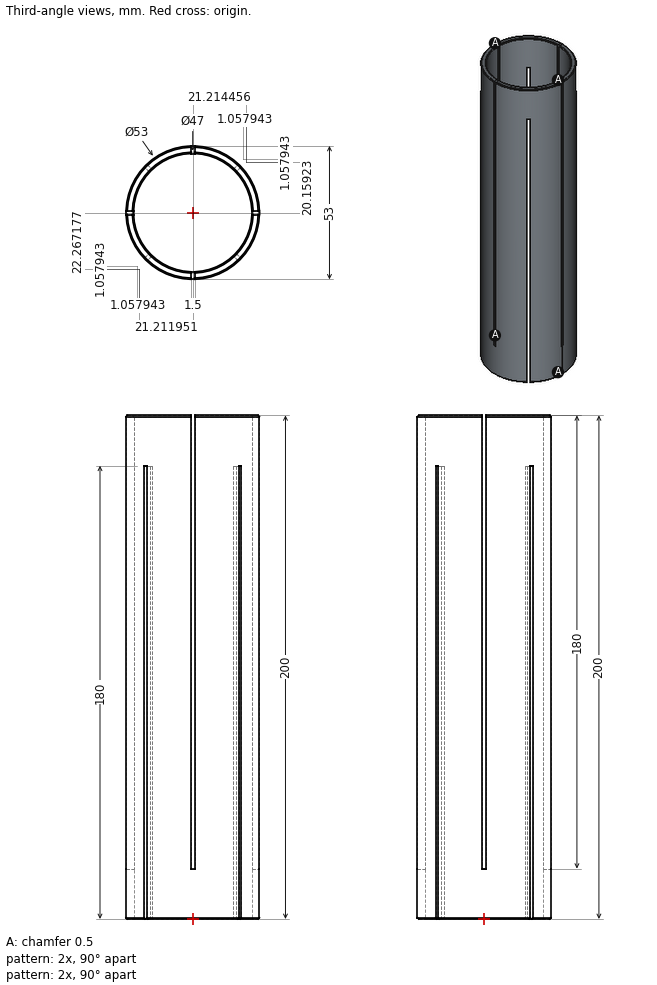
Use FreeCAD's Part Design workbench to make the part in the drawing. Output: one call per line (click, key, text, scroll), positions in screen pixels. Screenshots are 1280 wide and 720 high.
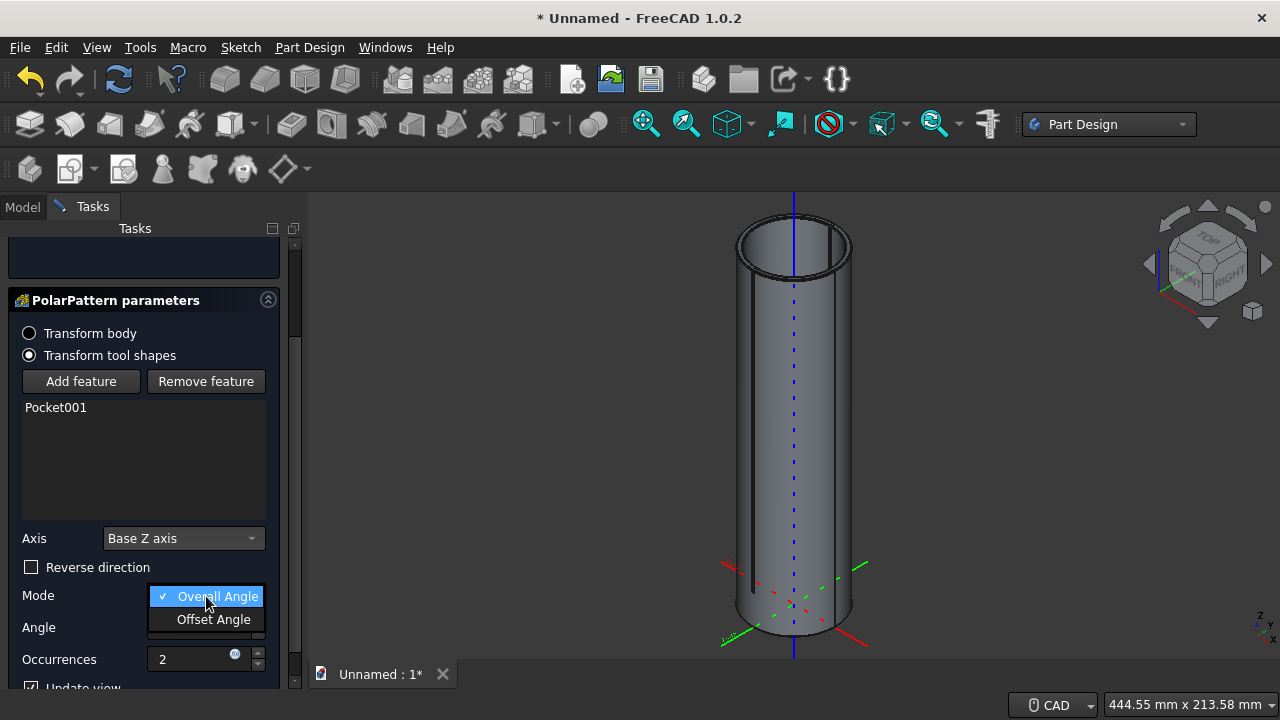
click(206, 620)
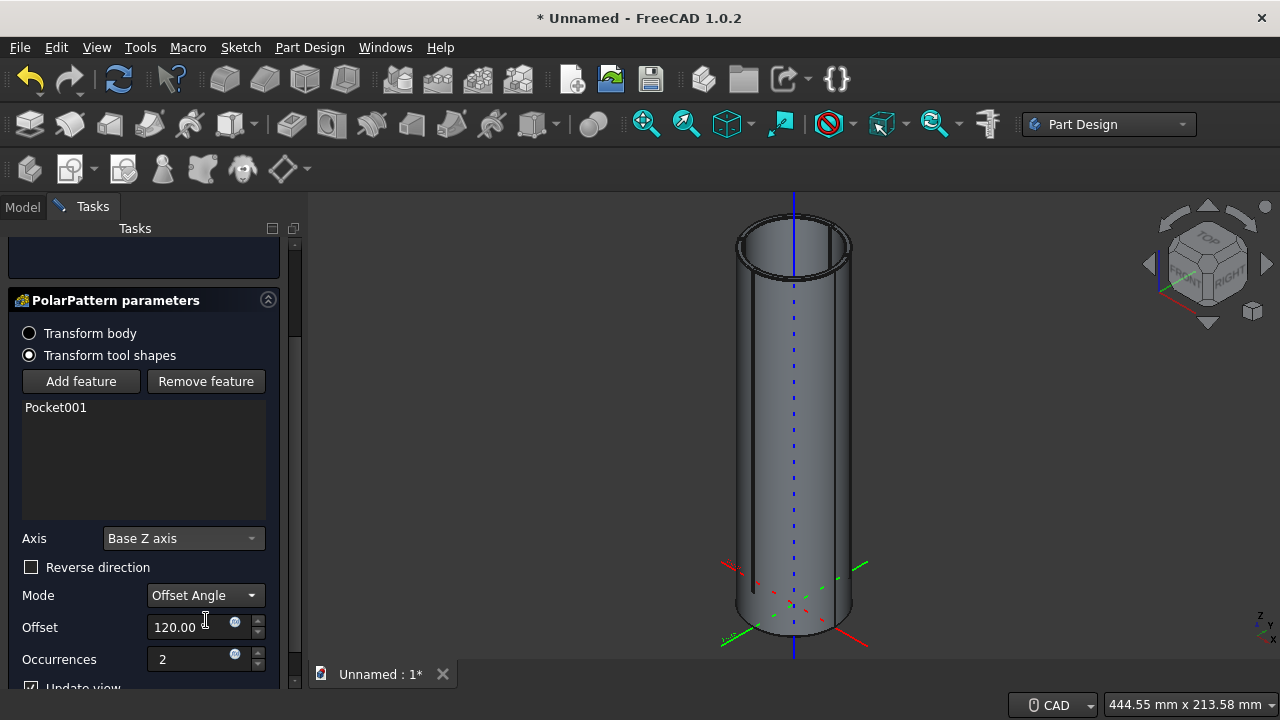
triple_click(198, 627)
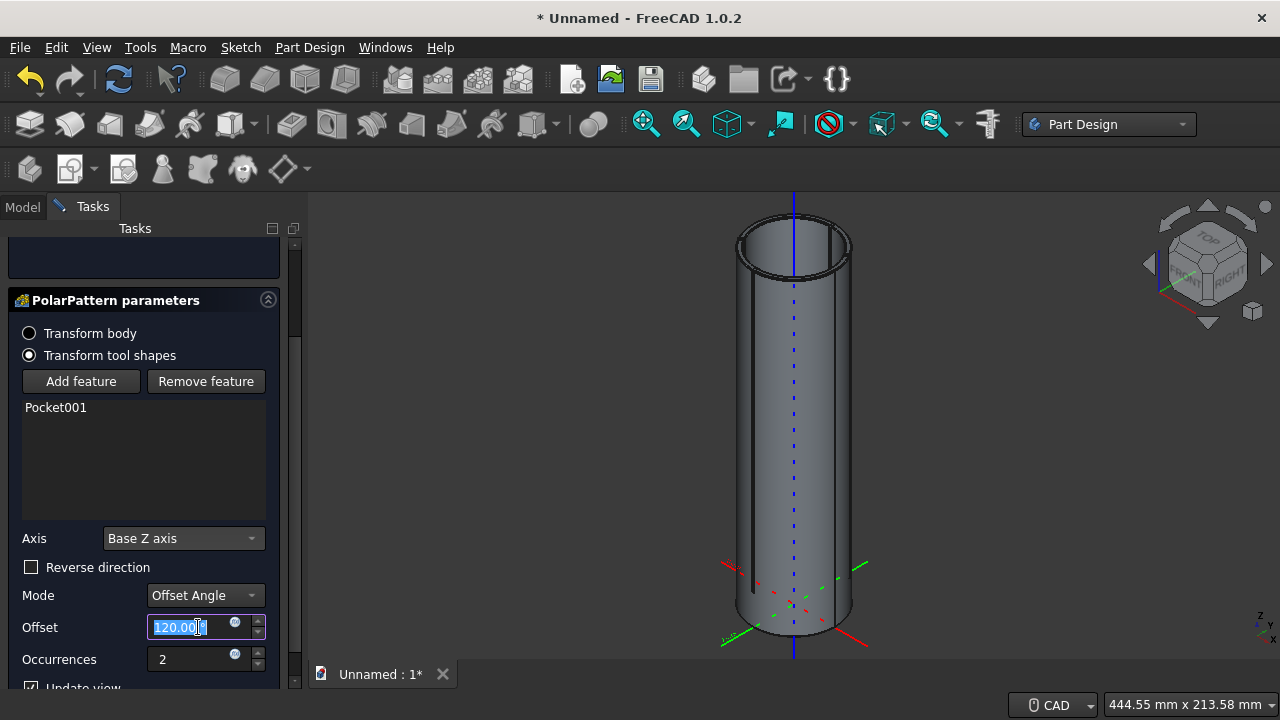
text(90)
key(Tab)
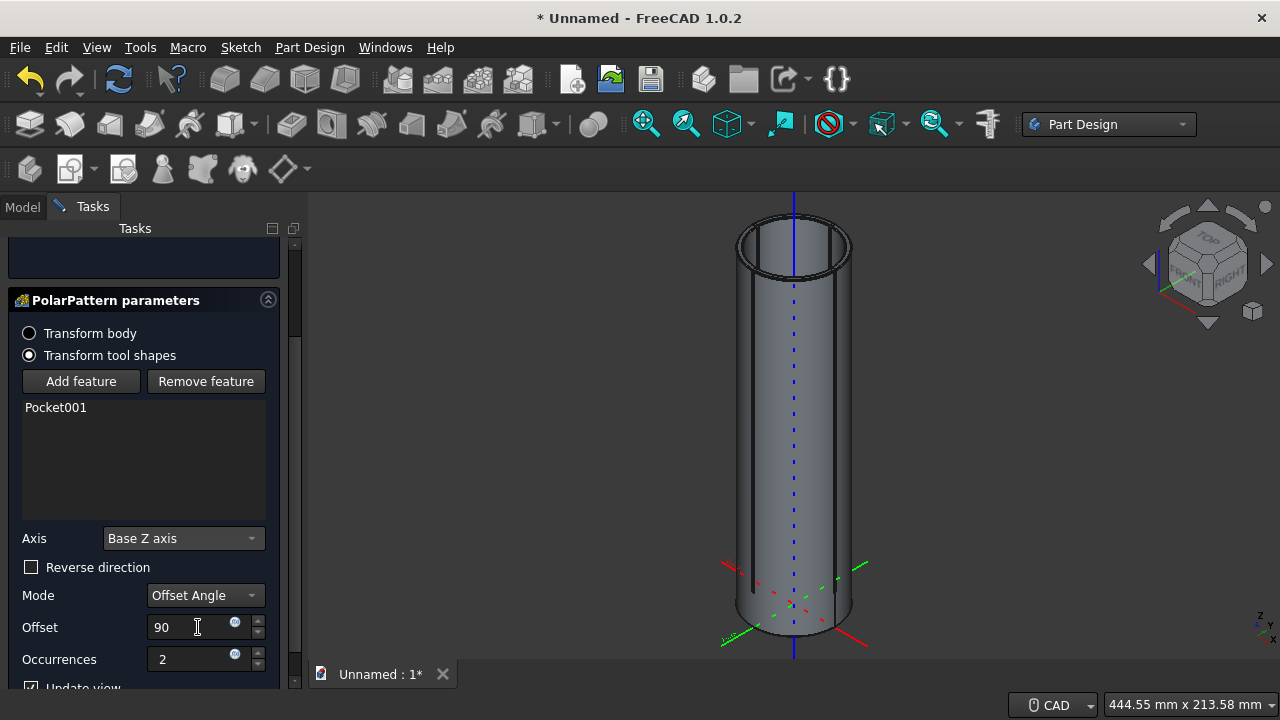
triple_click(198, 659)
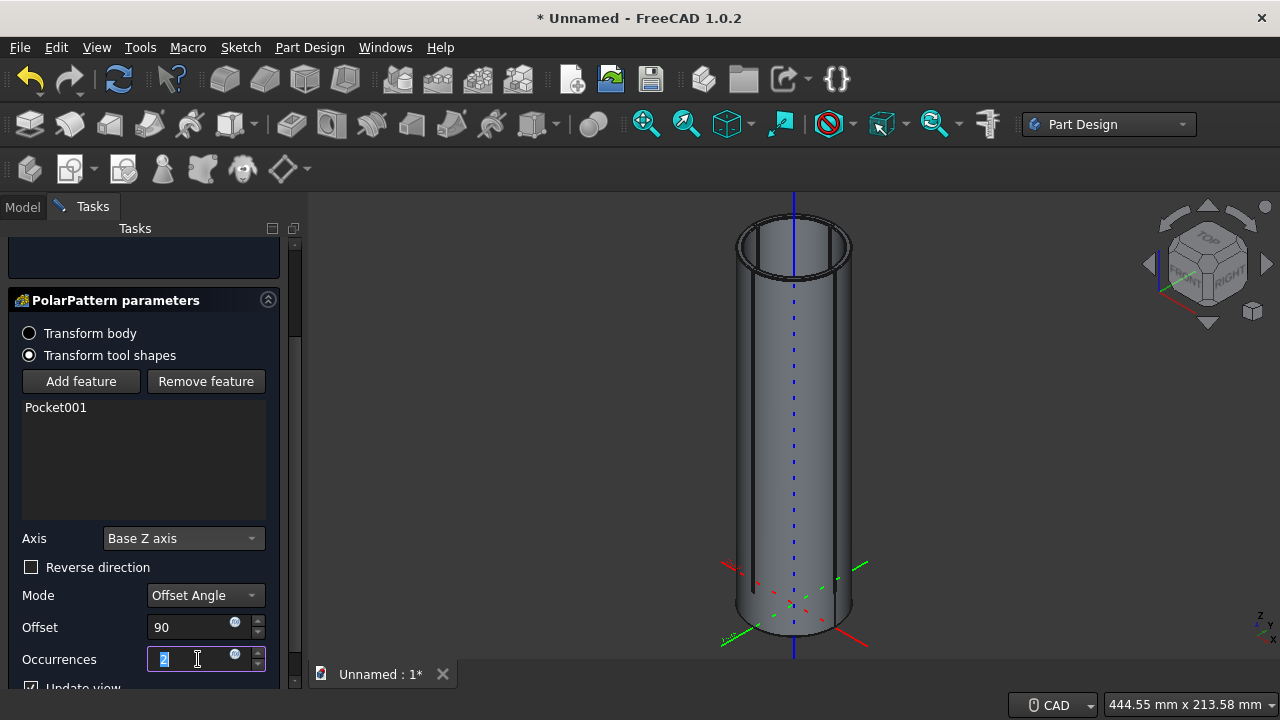
text(2)
key(Tab)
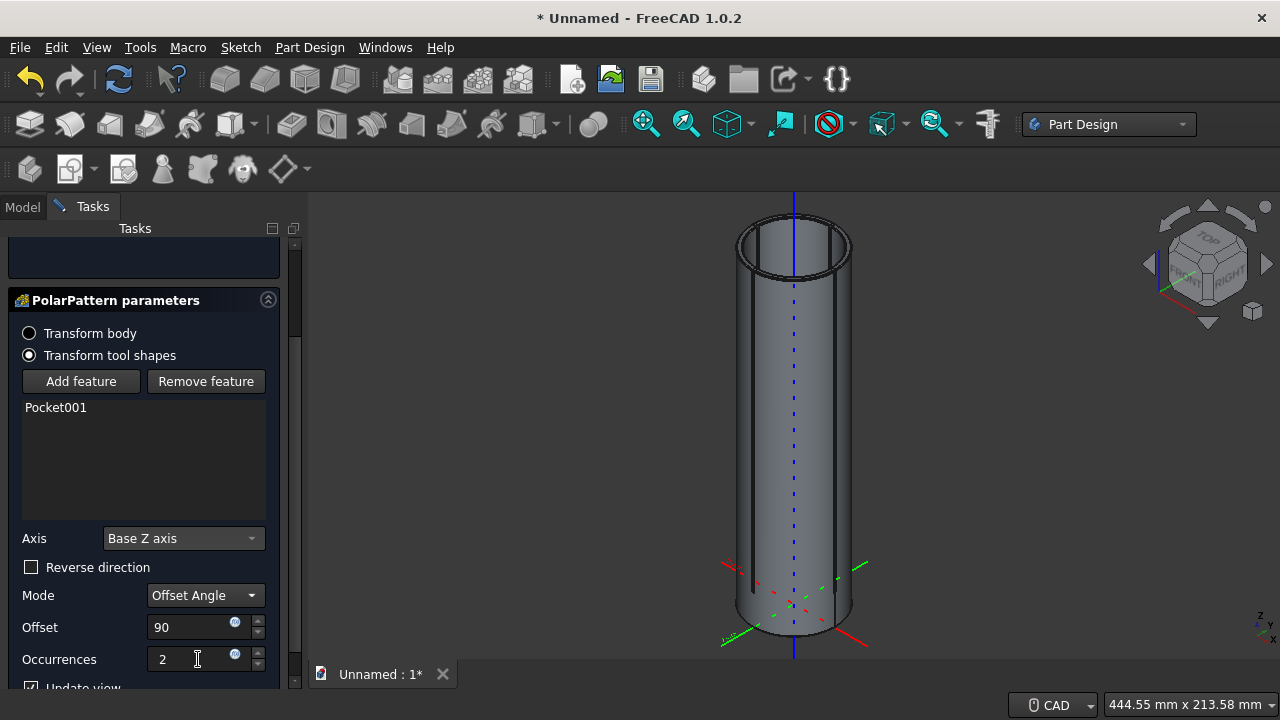
scroll(295, 463, up, 3)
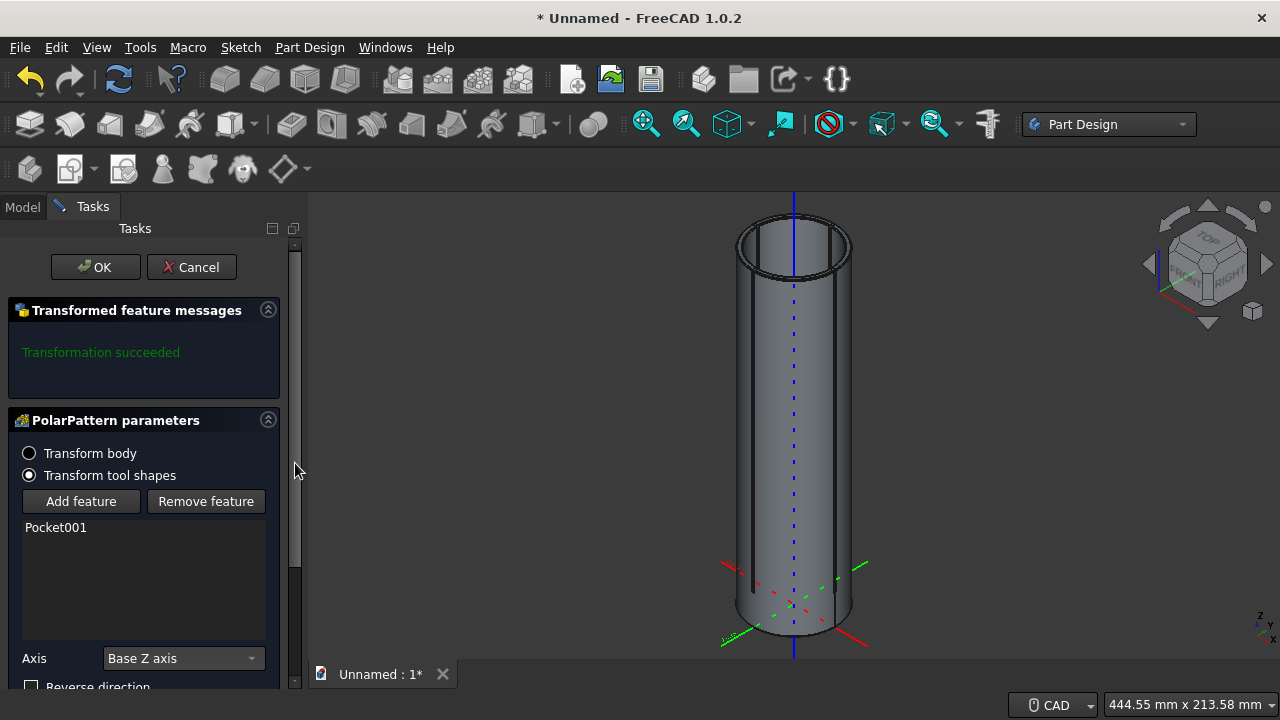
click(96, 267)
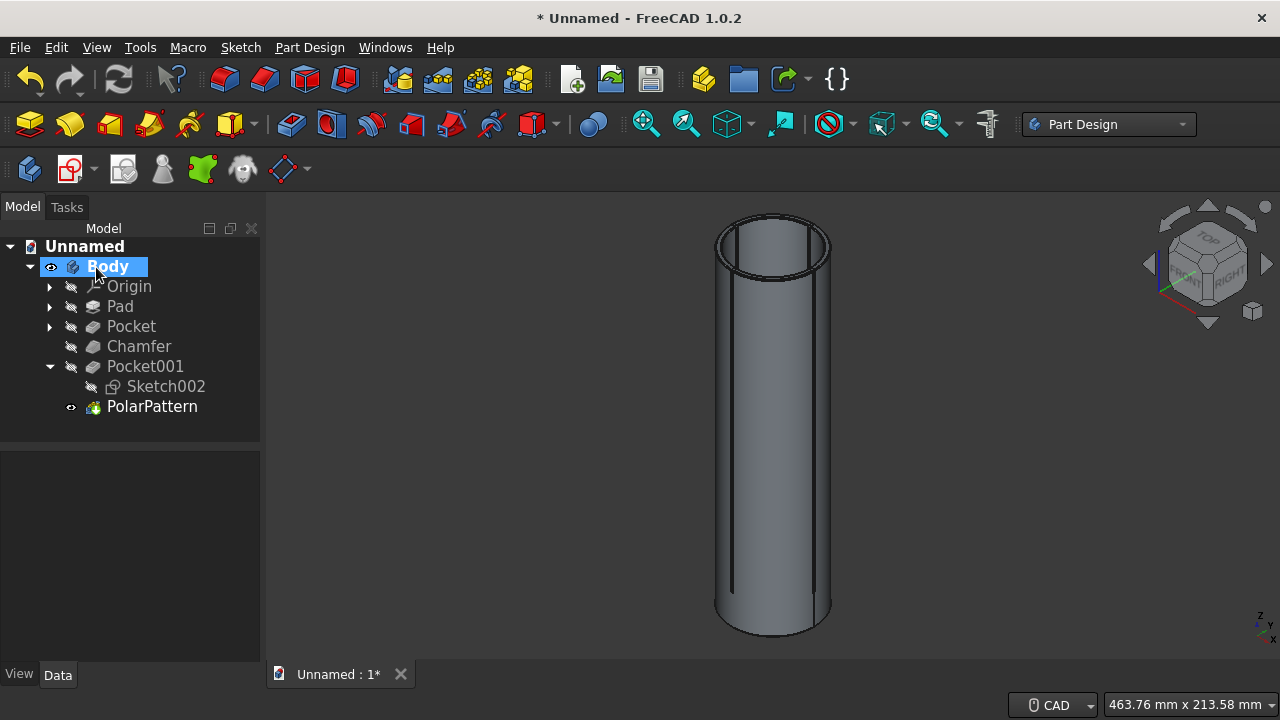
key(5)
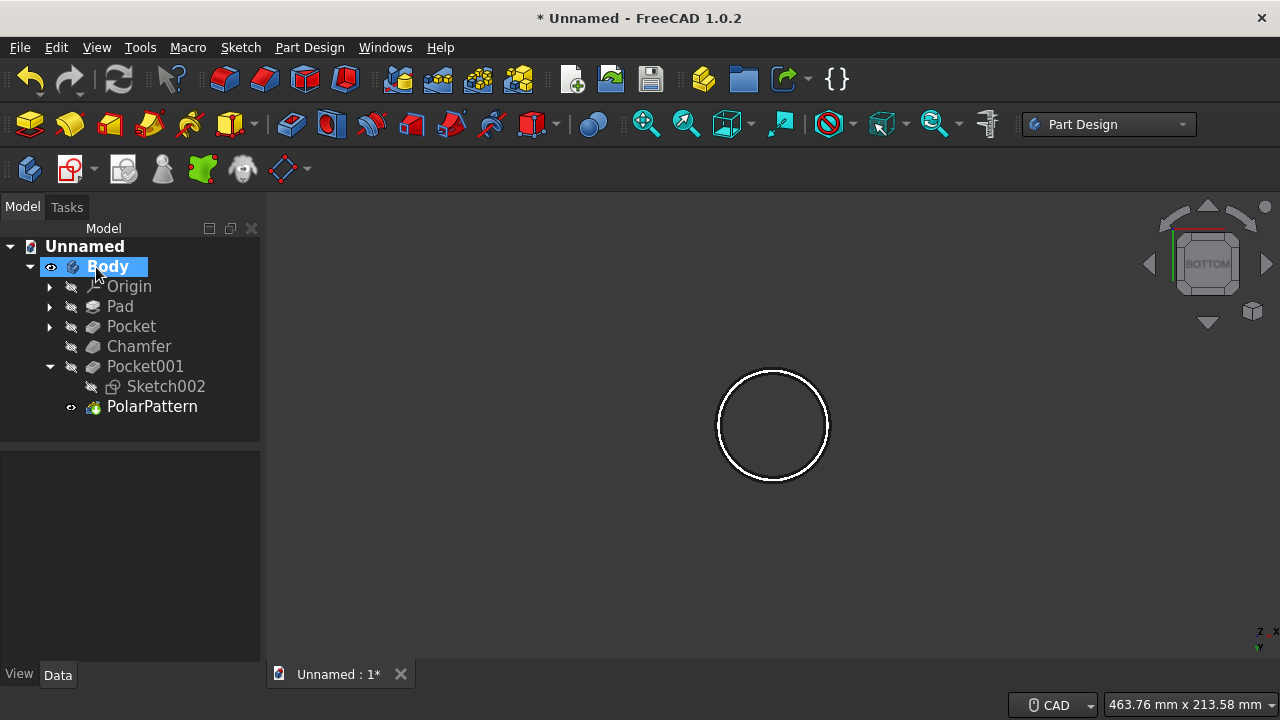
click(648, 124)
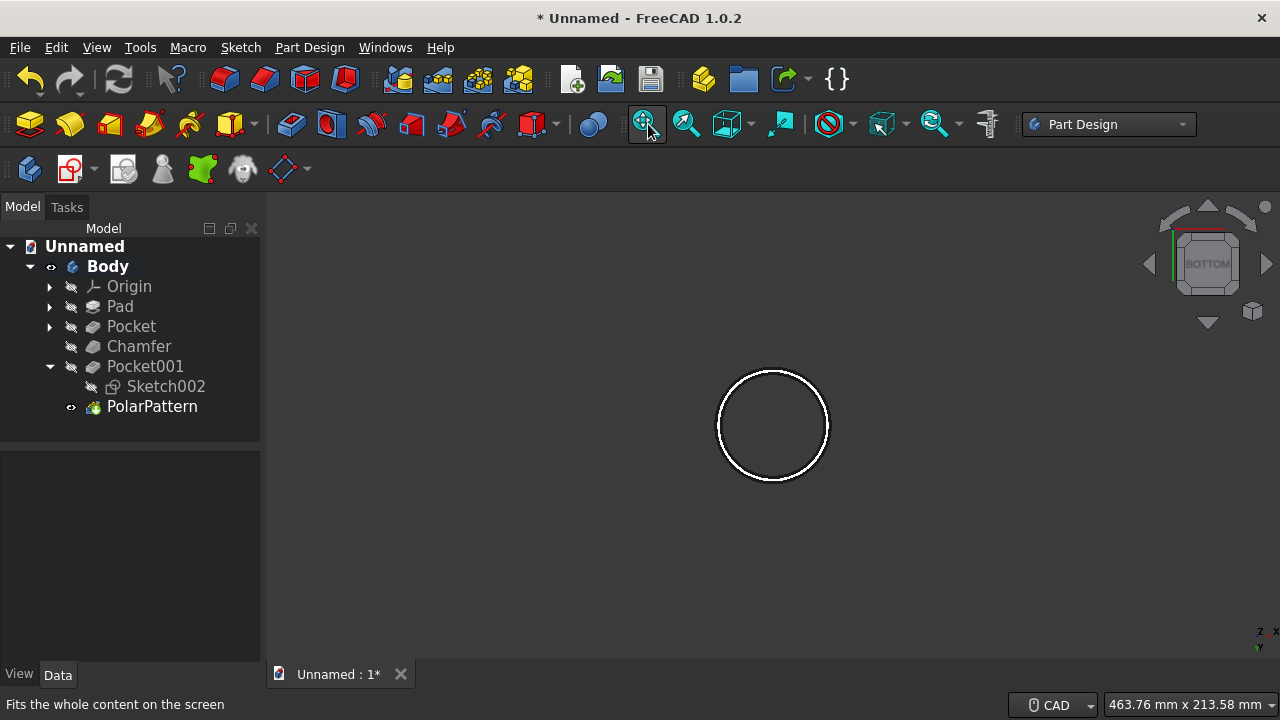
scroll(725, 396, up, 11)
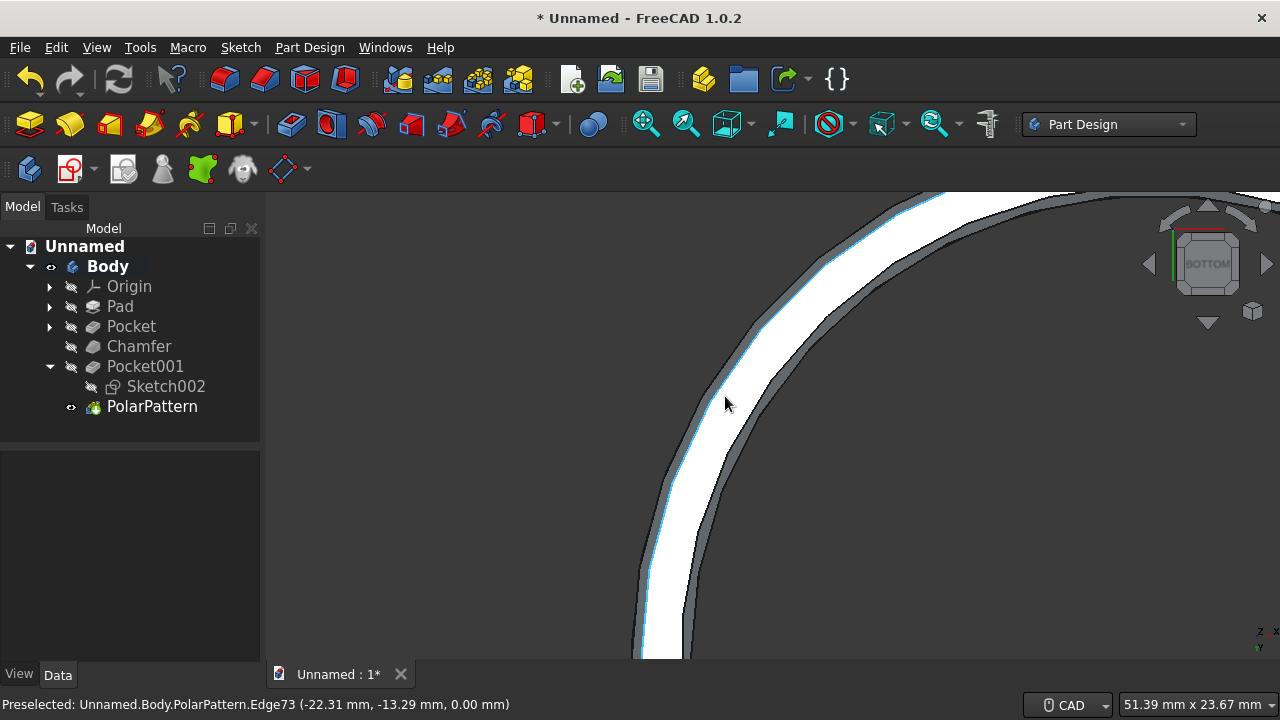
click(724, 404)